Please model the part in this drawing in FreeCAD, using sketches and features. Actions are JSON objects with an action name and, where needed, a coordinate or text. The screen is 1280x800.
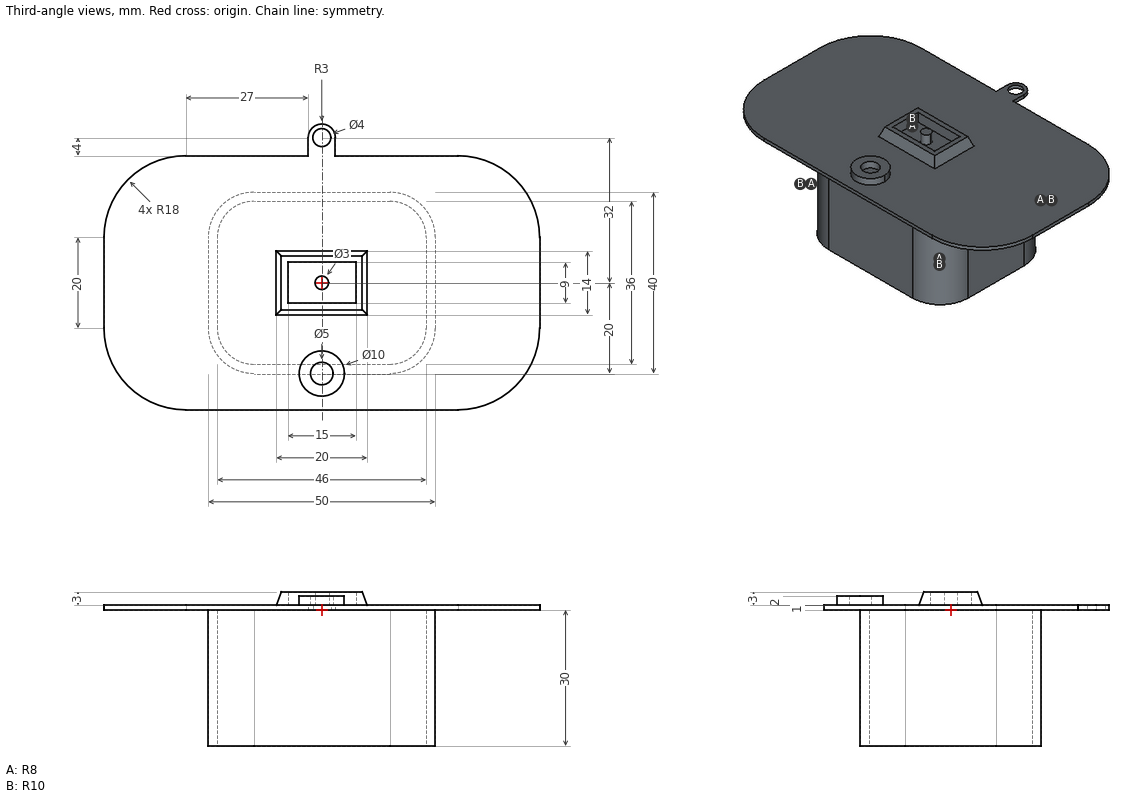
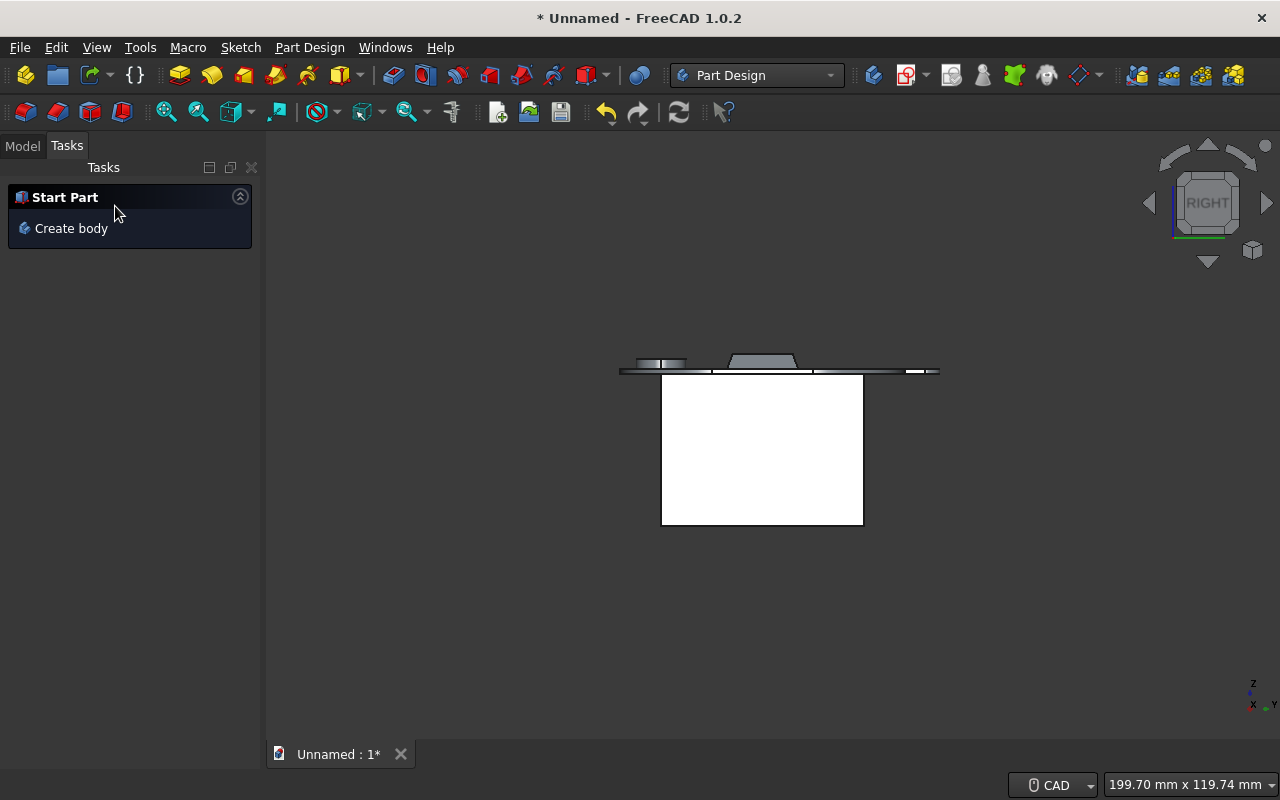
{"action": "left_click", "coordinate": [168, 112]}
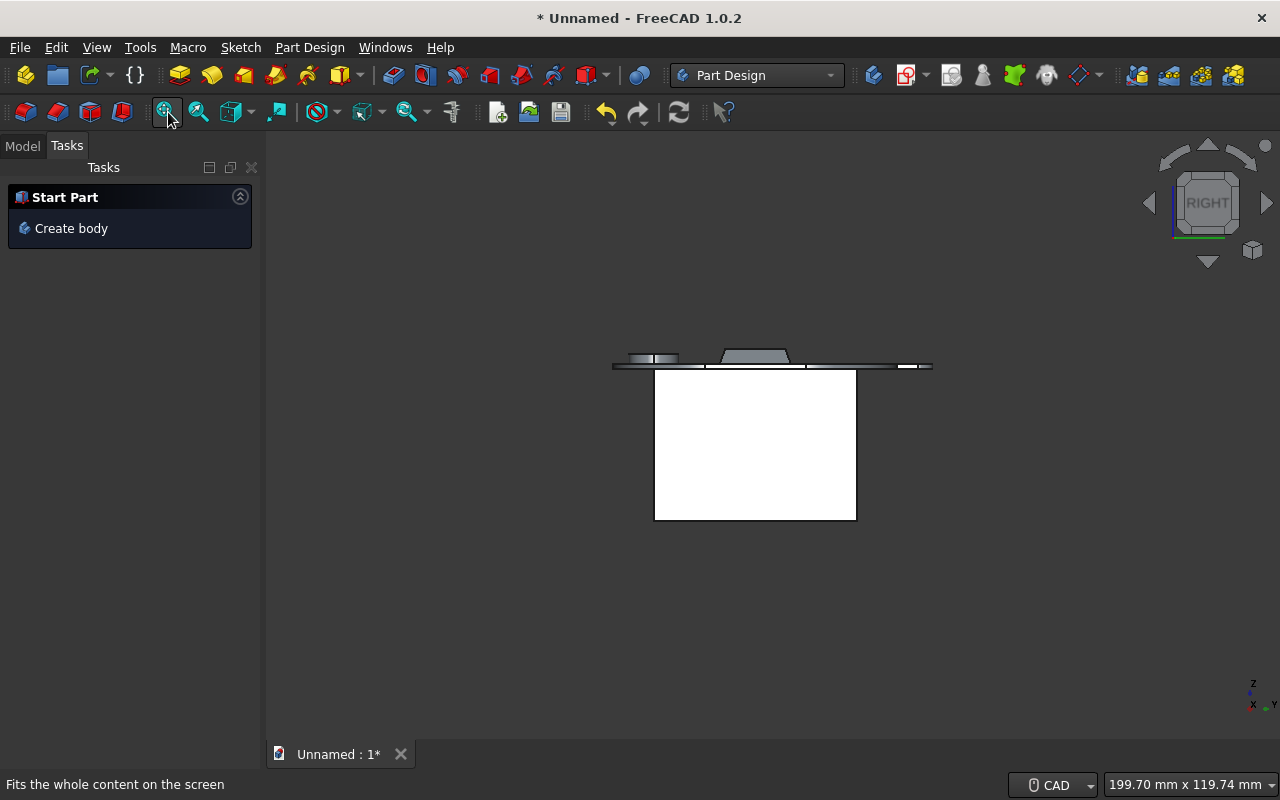
{"action": "key", "text": "5"}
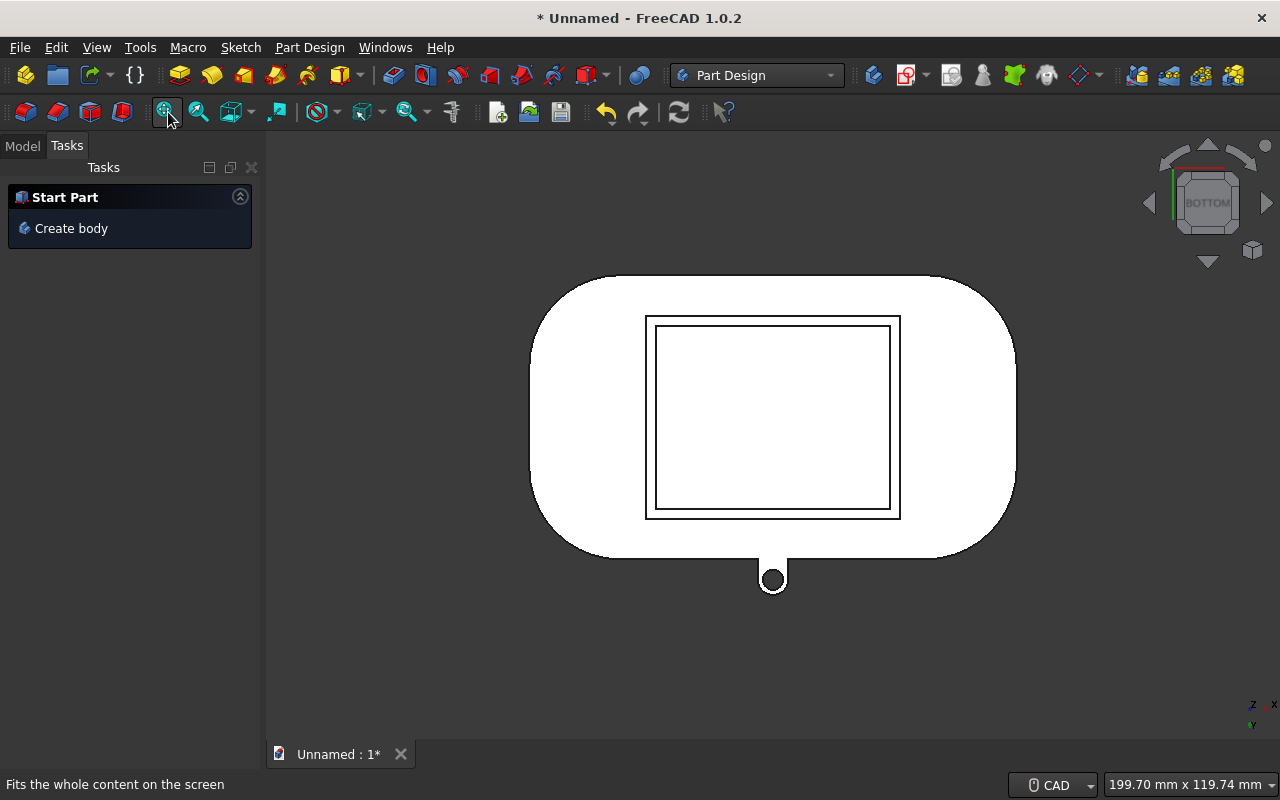
{"action": "key", "text": "4"}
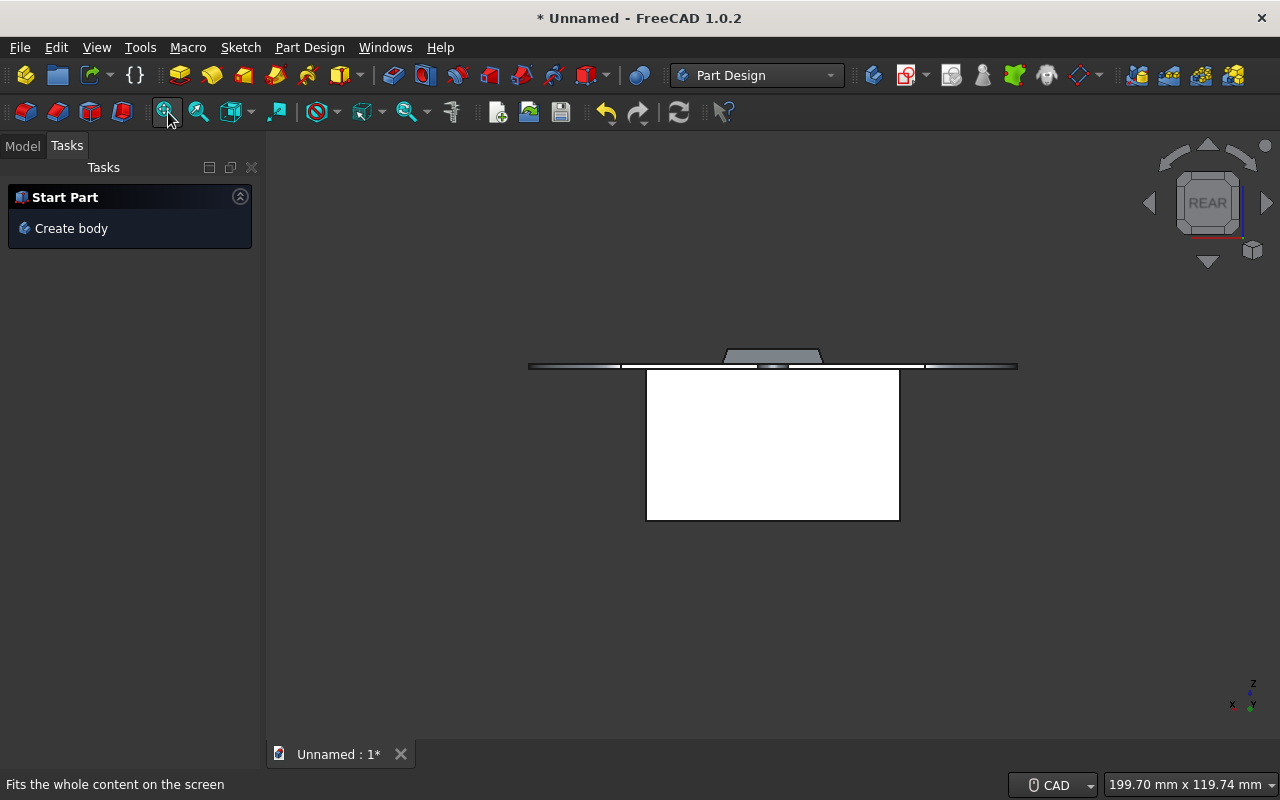
{"action": "key", "text": "6"}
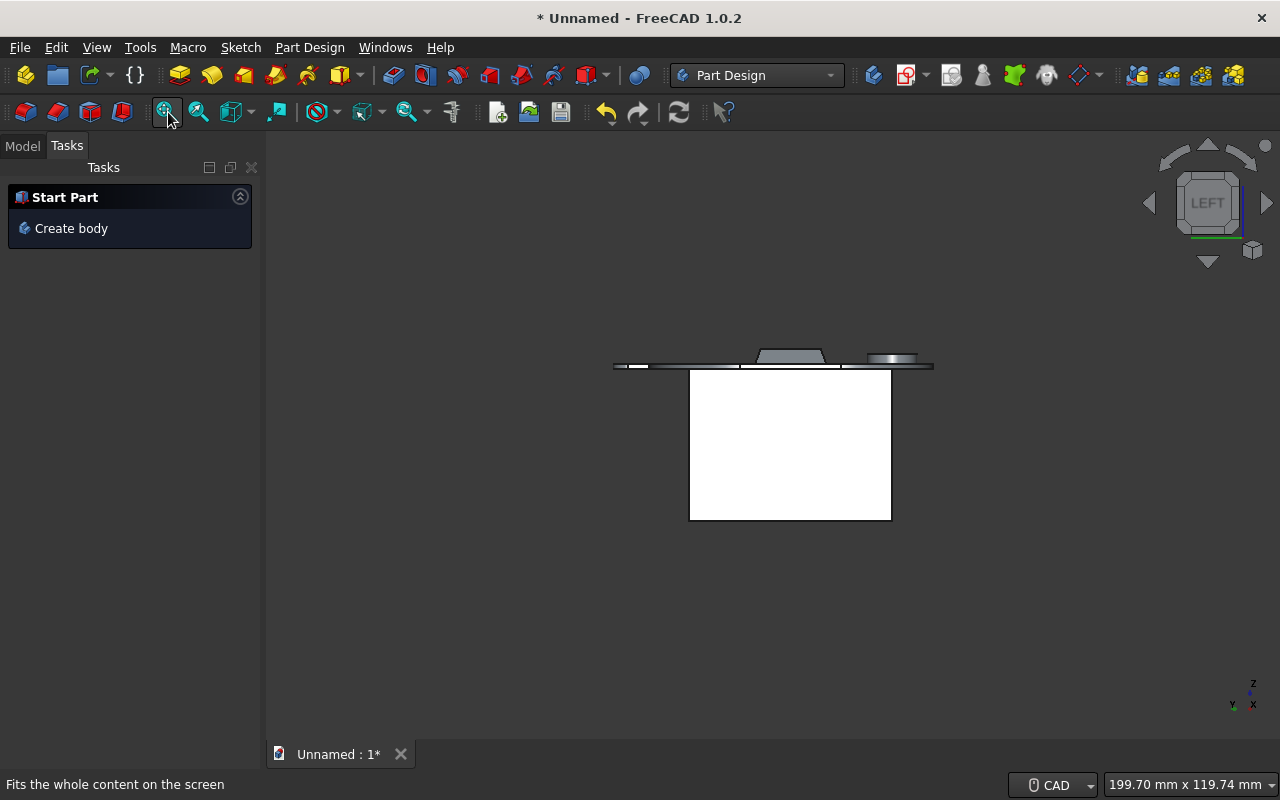
{"action": "left_click", "coordinate": [168, 112]}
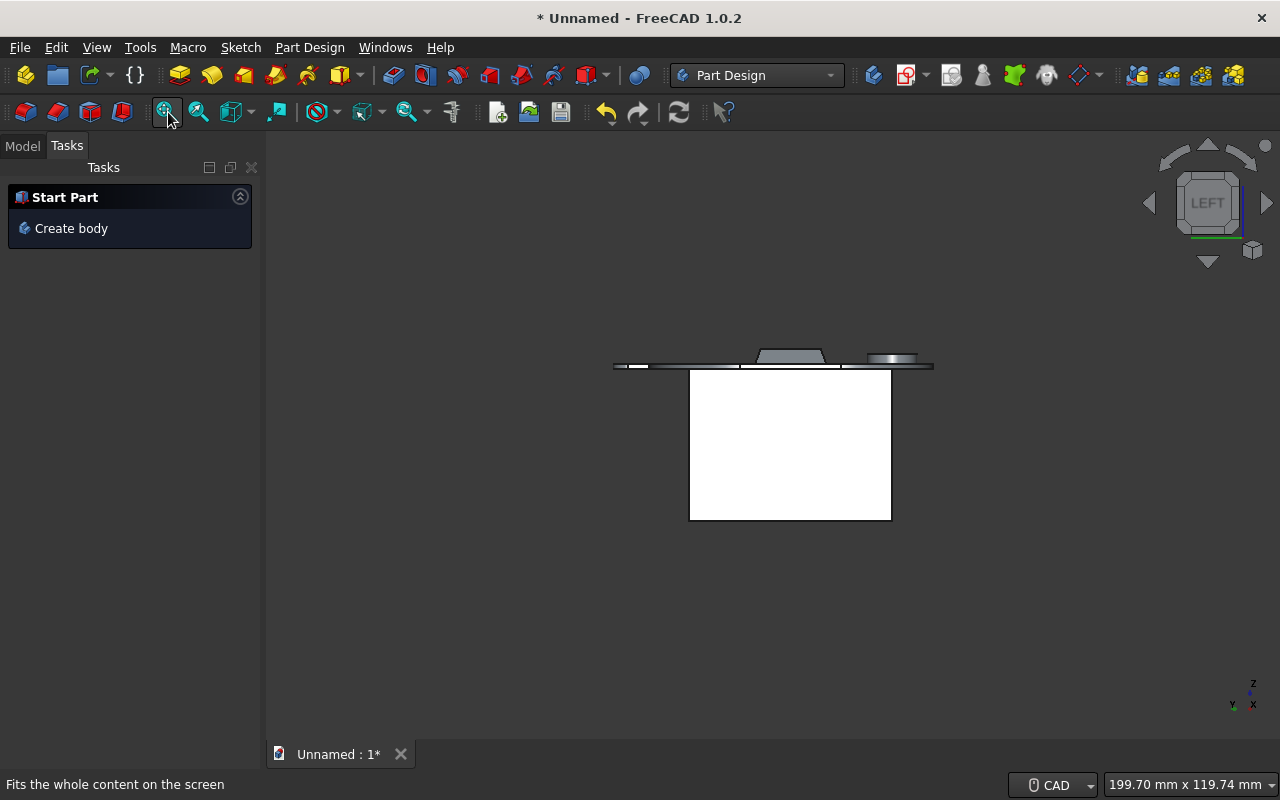
{"action": "key", "text": "v 3"}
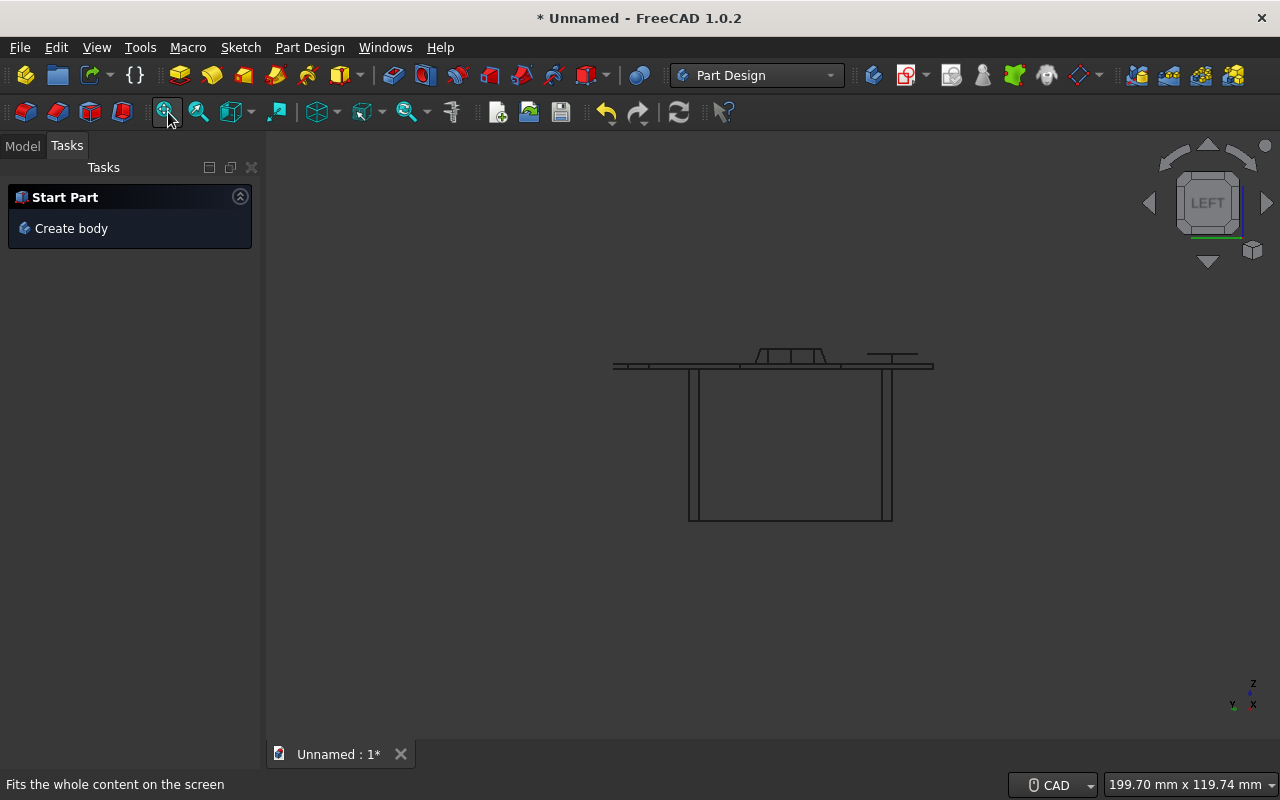
{"action": "key", "text": "0"}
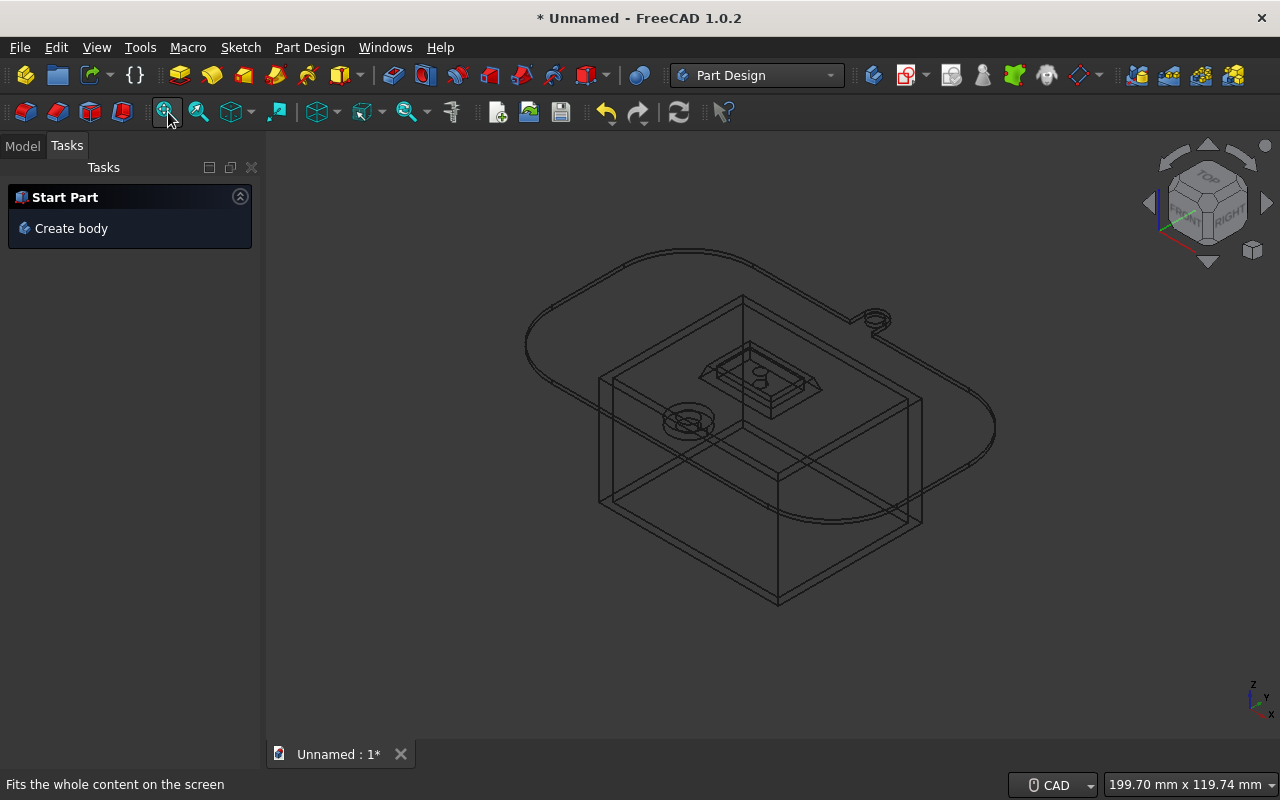
{"action": "left_click", "coordinate": [743, 327]}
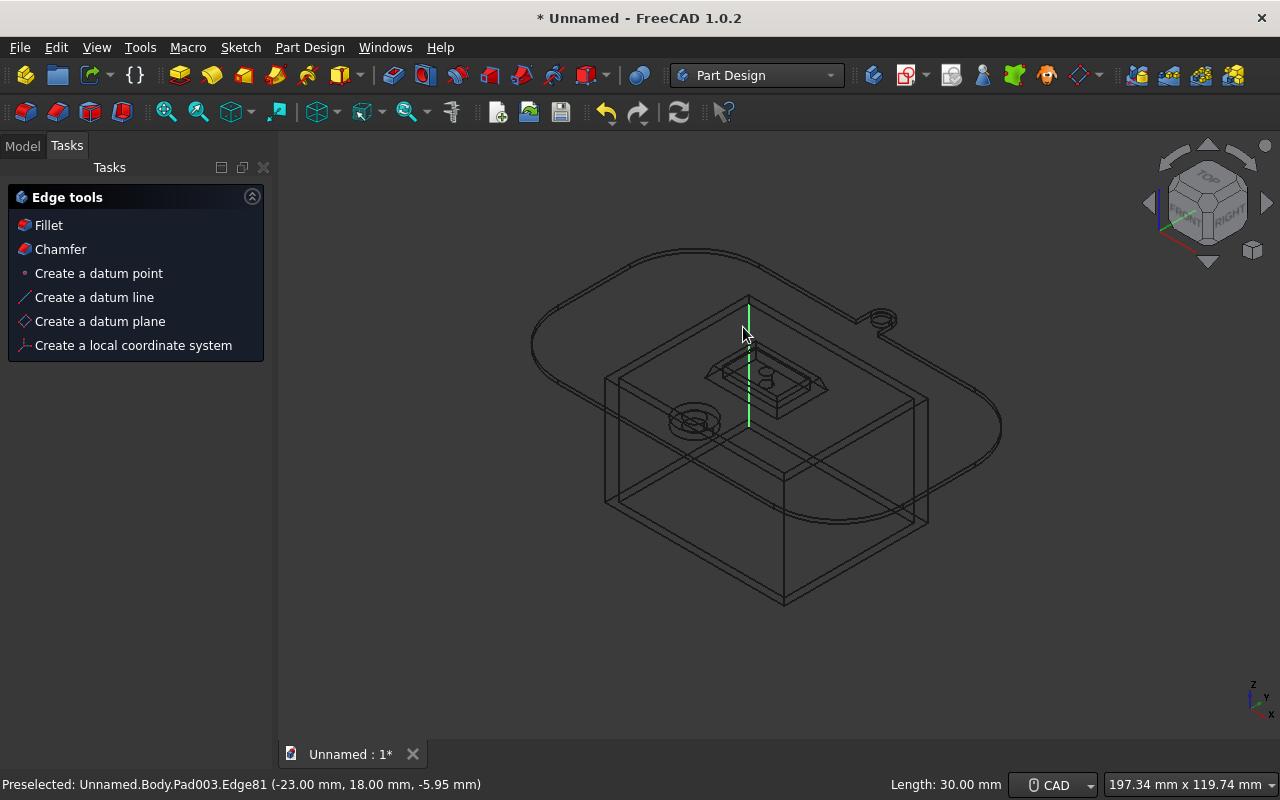
{"action": "left_click", "coordinate": [914, 460], "text": "ctrl"}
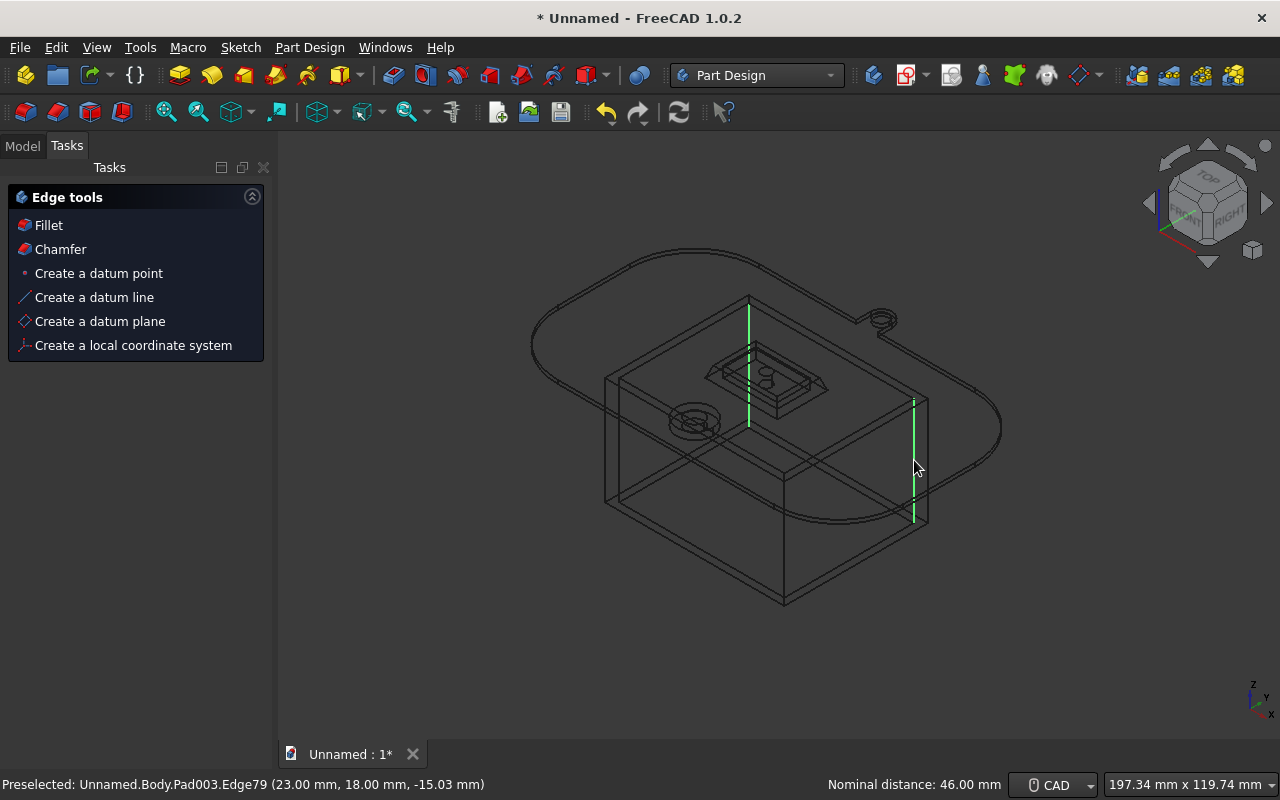
{"action": "left_click", "coordinate": [619, 439], "text": "ctrl"}